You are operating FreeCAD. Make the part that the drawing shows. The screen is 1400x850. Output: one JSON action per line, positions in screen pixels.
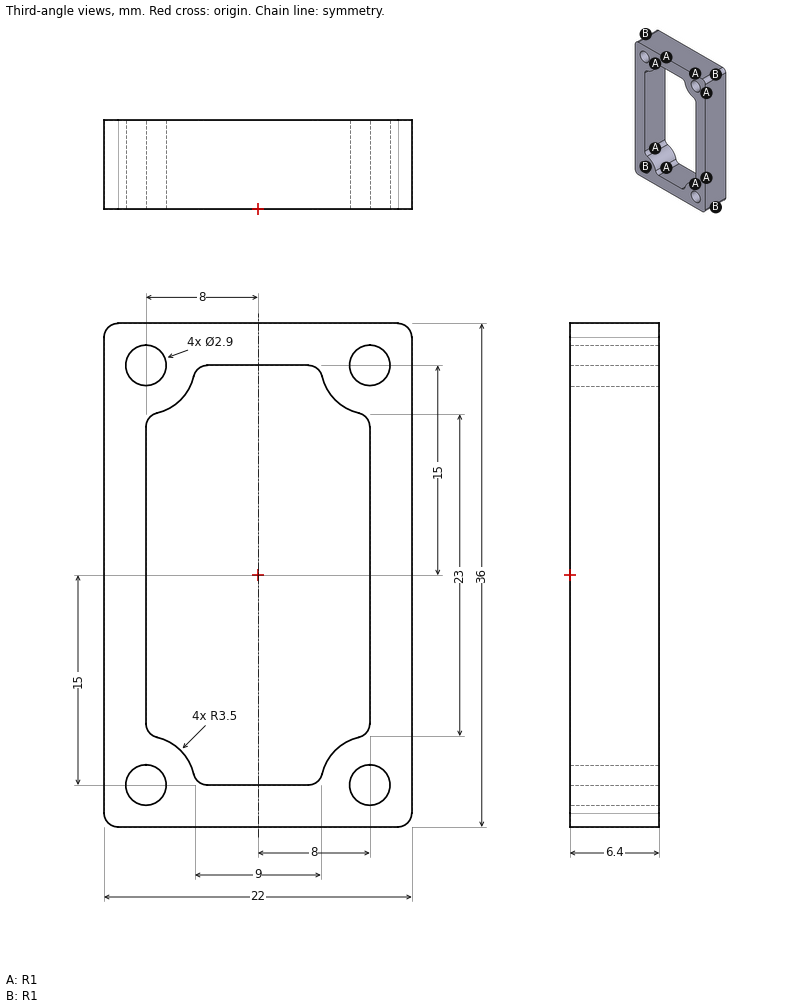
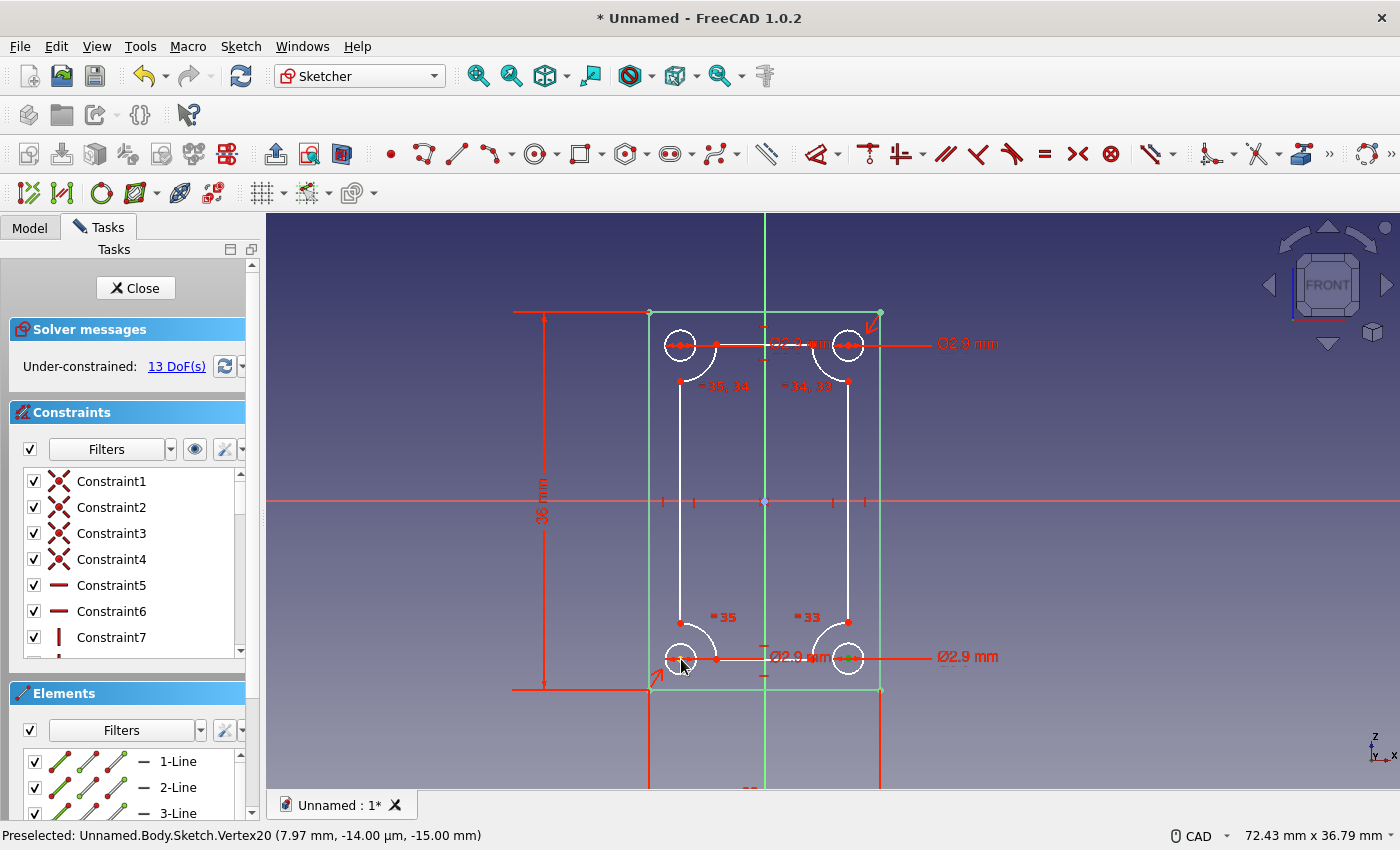
{"action": "left_click", "coordinate": [848, 346]}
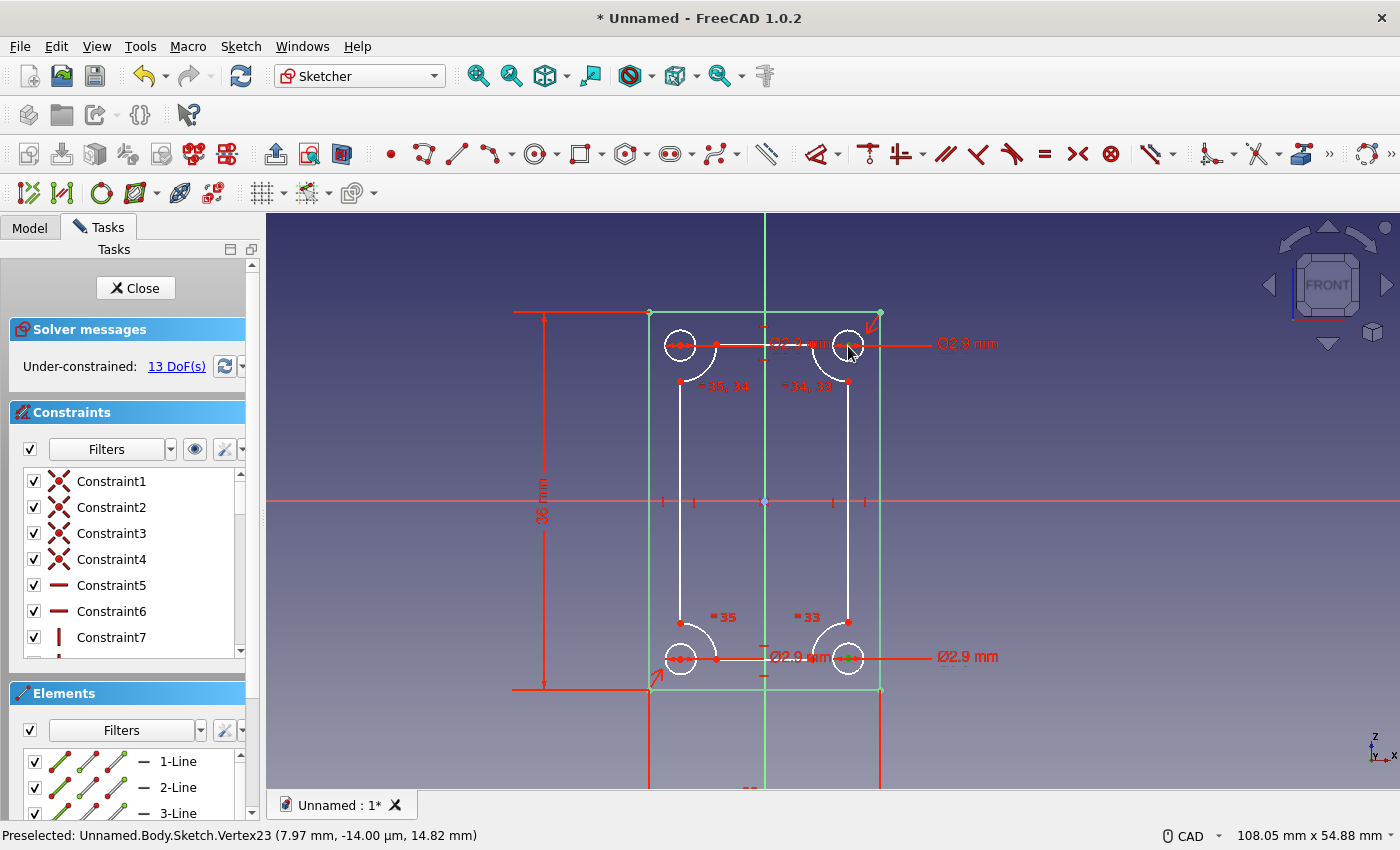
{"action": "left_click", "coordinate": [361, 501]}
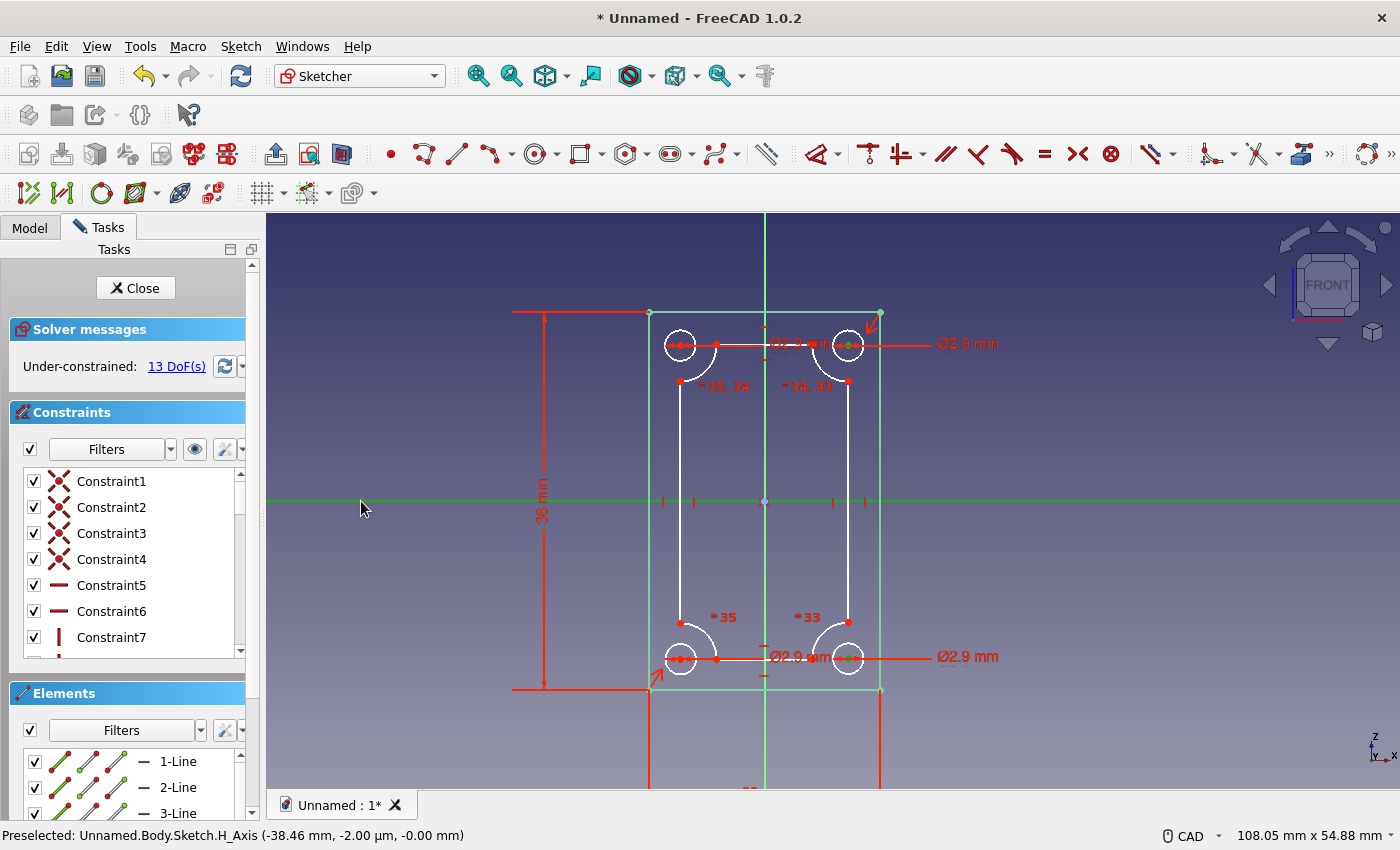
{"action": "left_click", "coordinate": [1078, 154]}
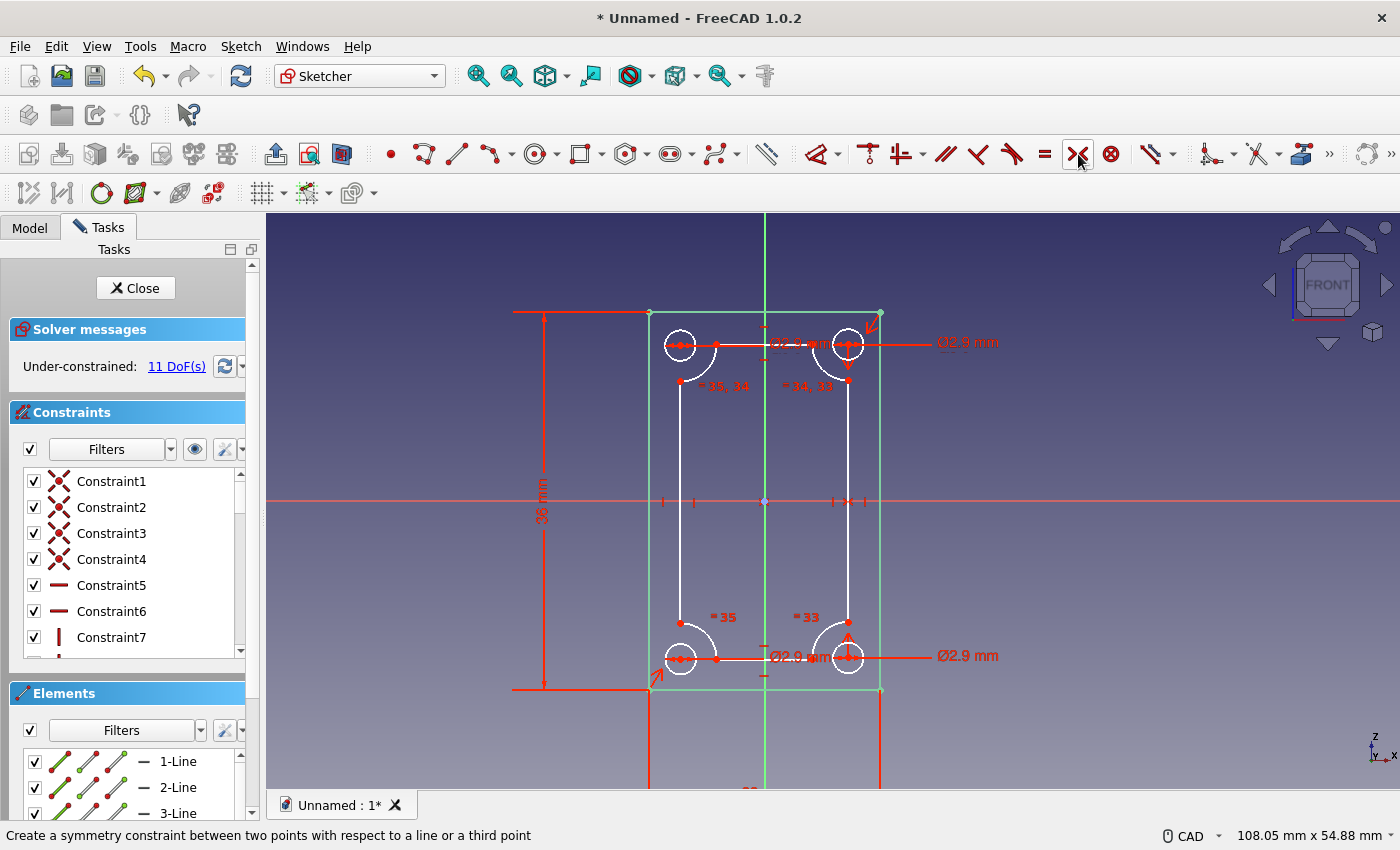
{"action": "left_click", "coordinate": [848, 345]}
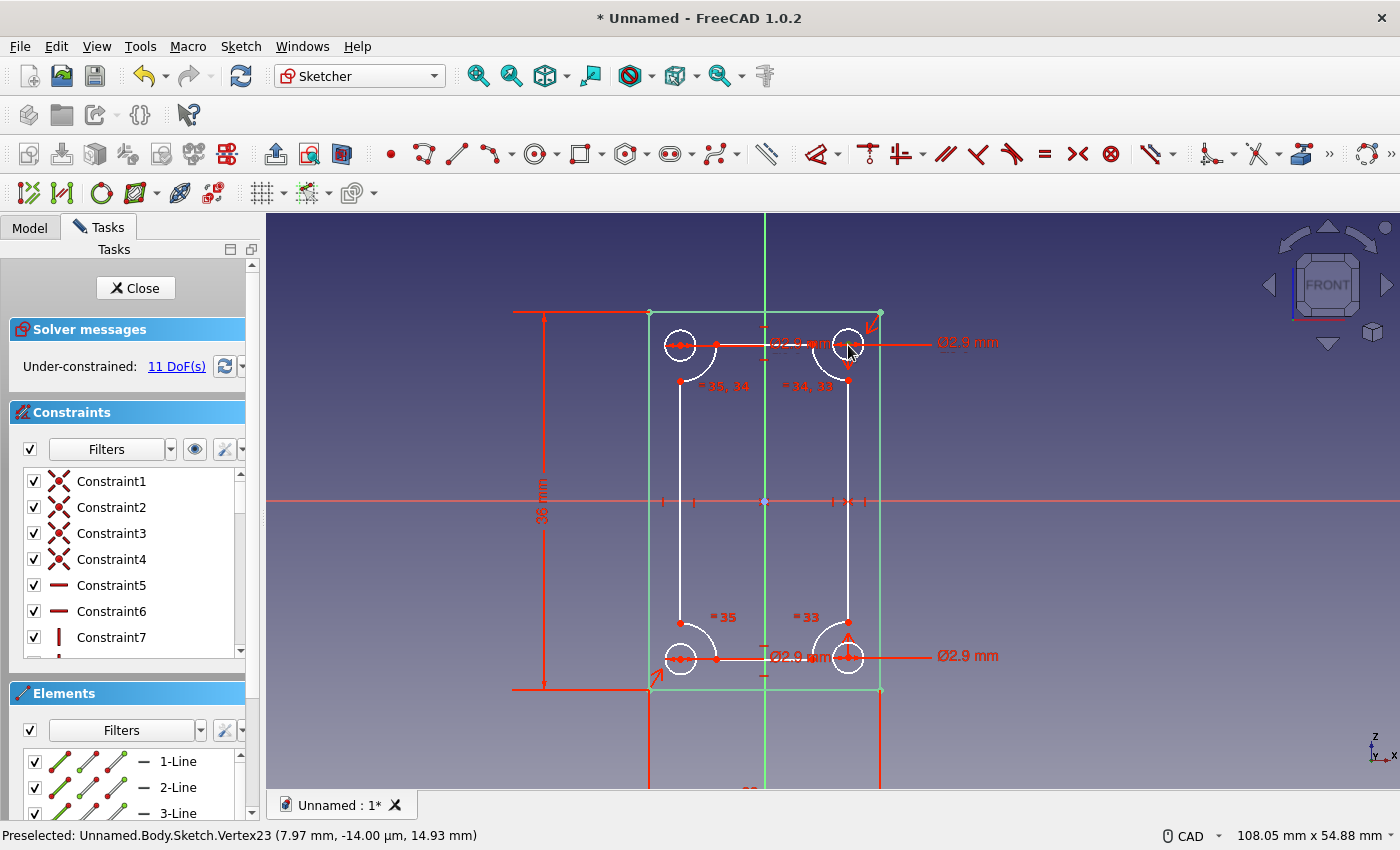
{"action": "left_click", "coordinate": [680, 346]}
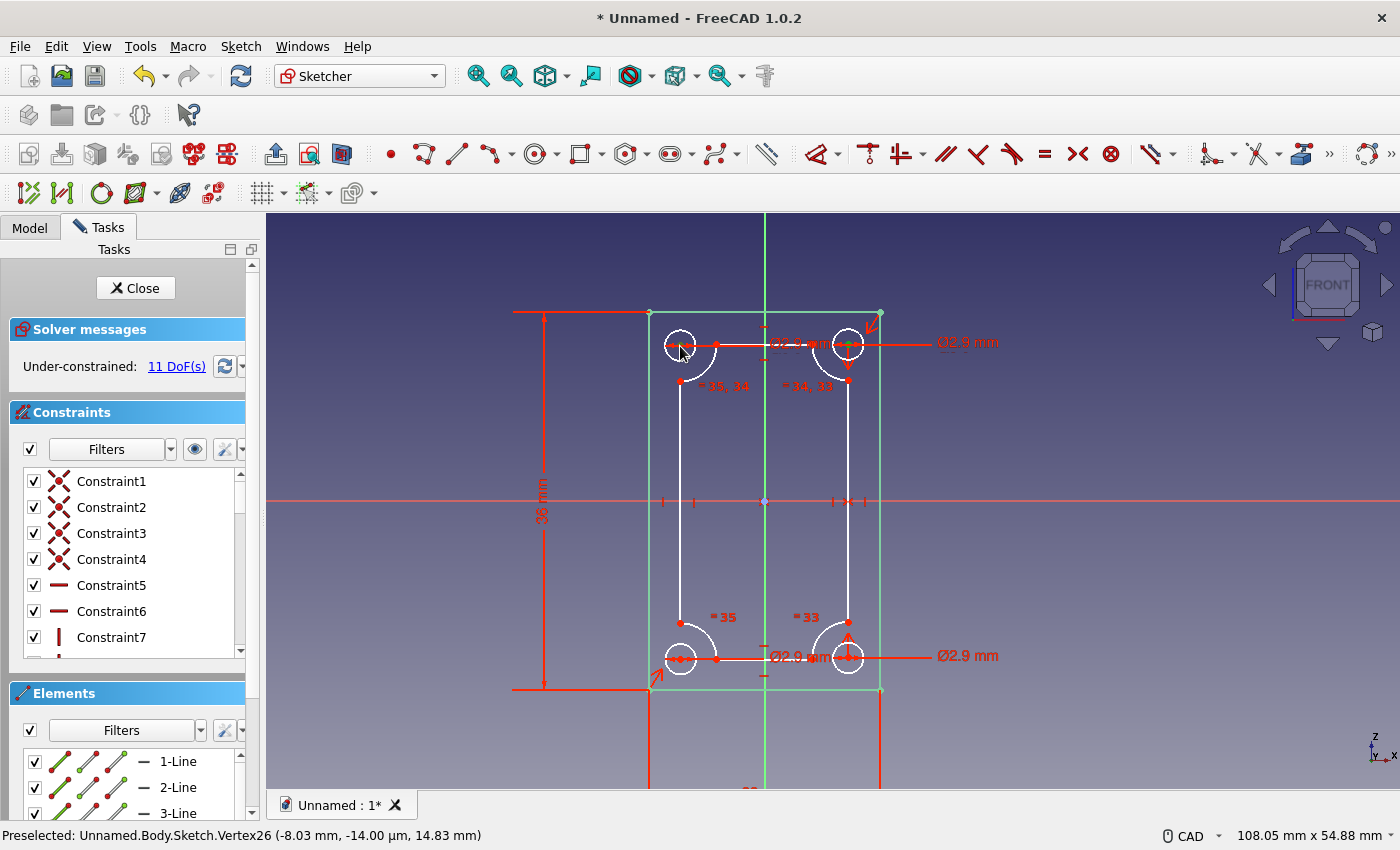
{"action": "left_click", "coordinate": [765, 724]}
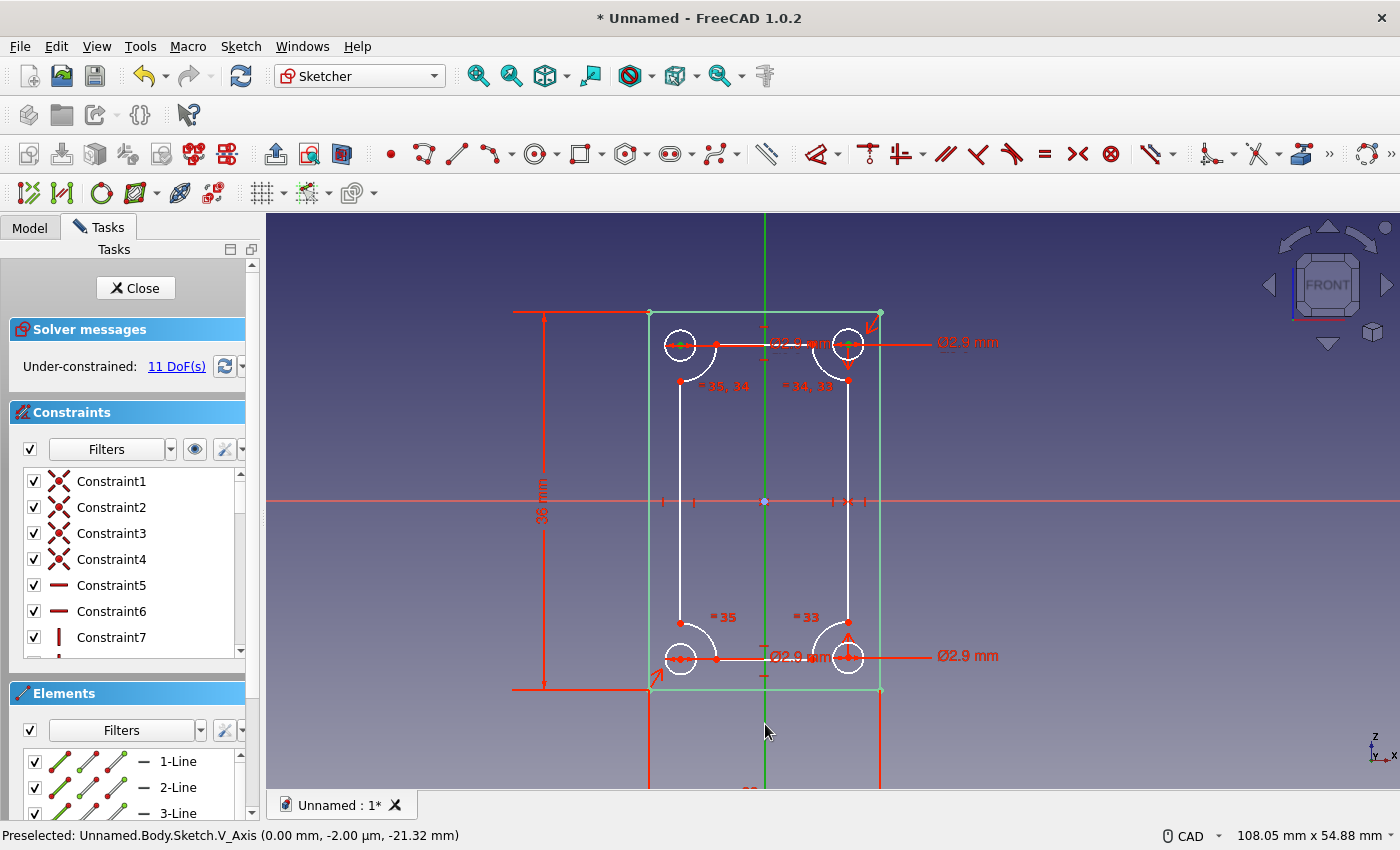
{"action": "left_click", "coordinate": [1078, 154]}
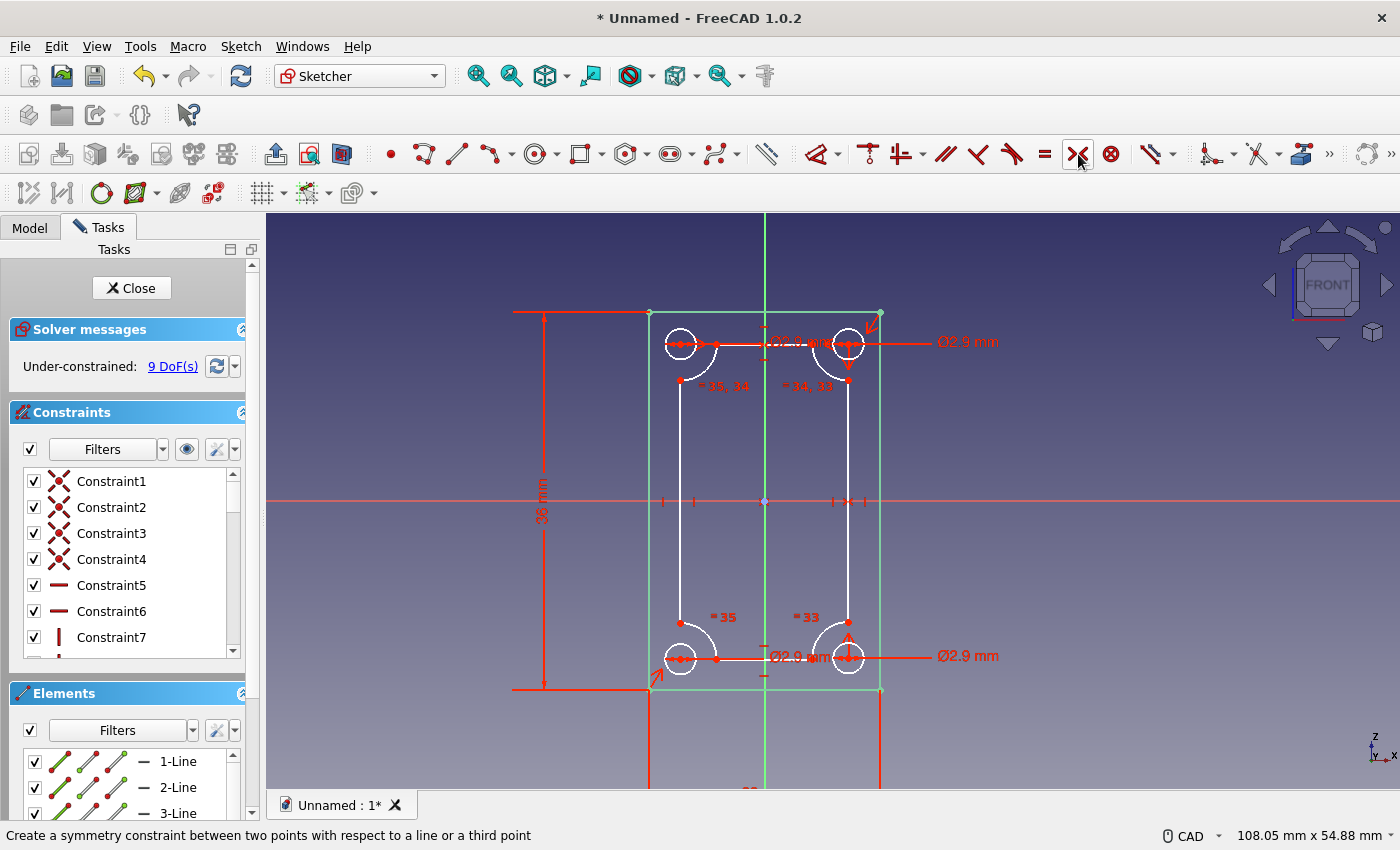
{"action": "left_click", "coordinate": [849, 658]}